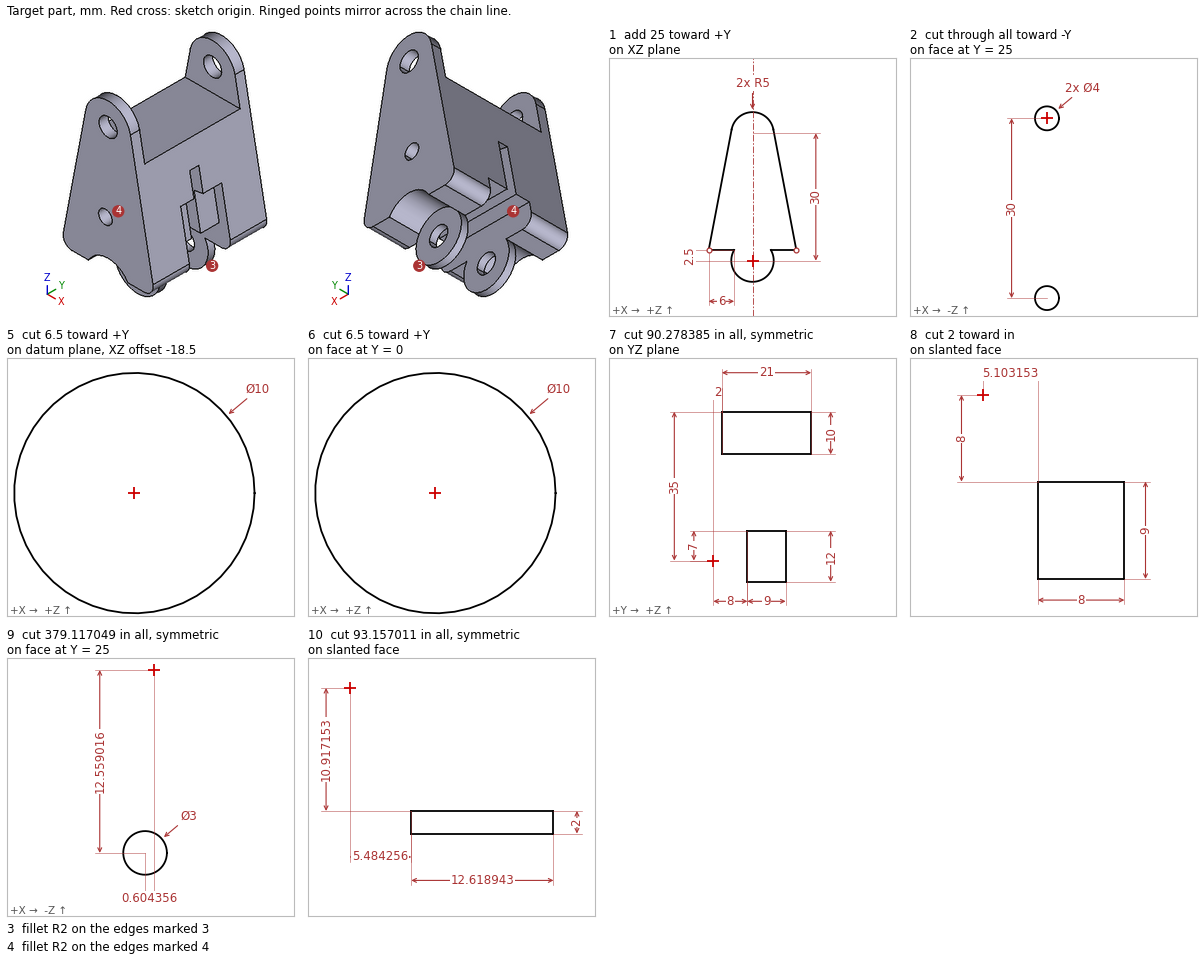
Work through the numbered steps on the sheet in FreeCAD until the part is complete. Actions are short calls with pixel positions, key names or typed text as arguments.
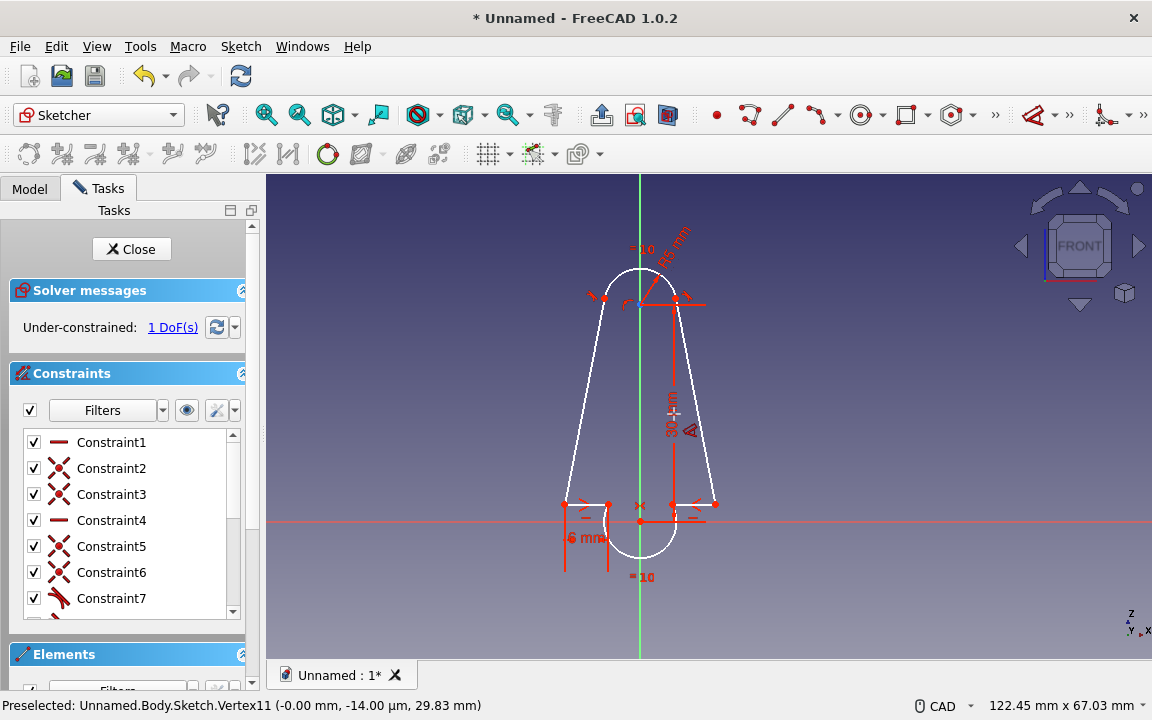
scroll(608, 505, up, 4)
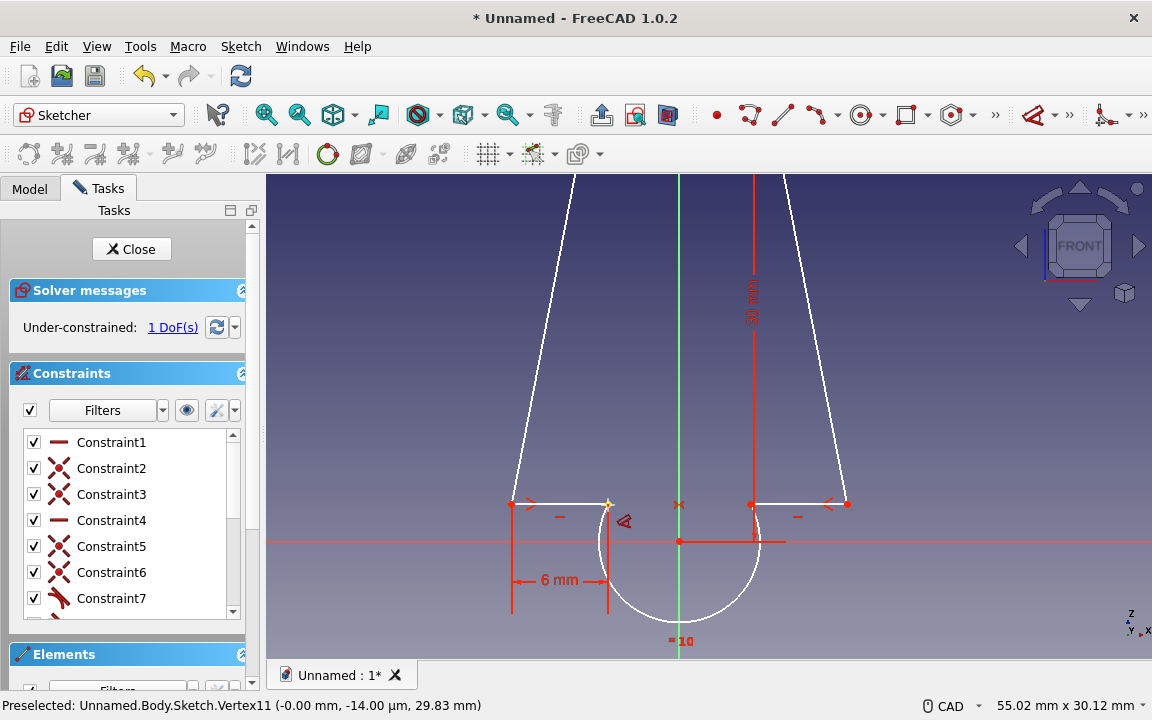
click(608, 504)
click(574, 523)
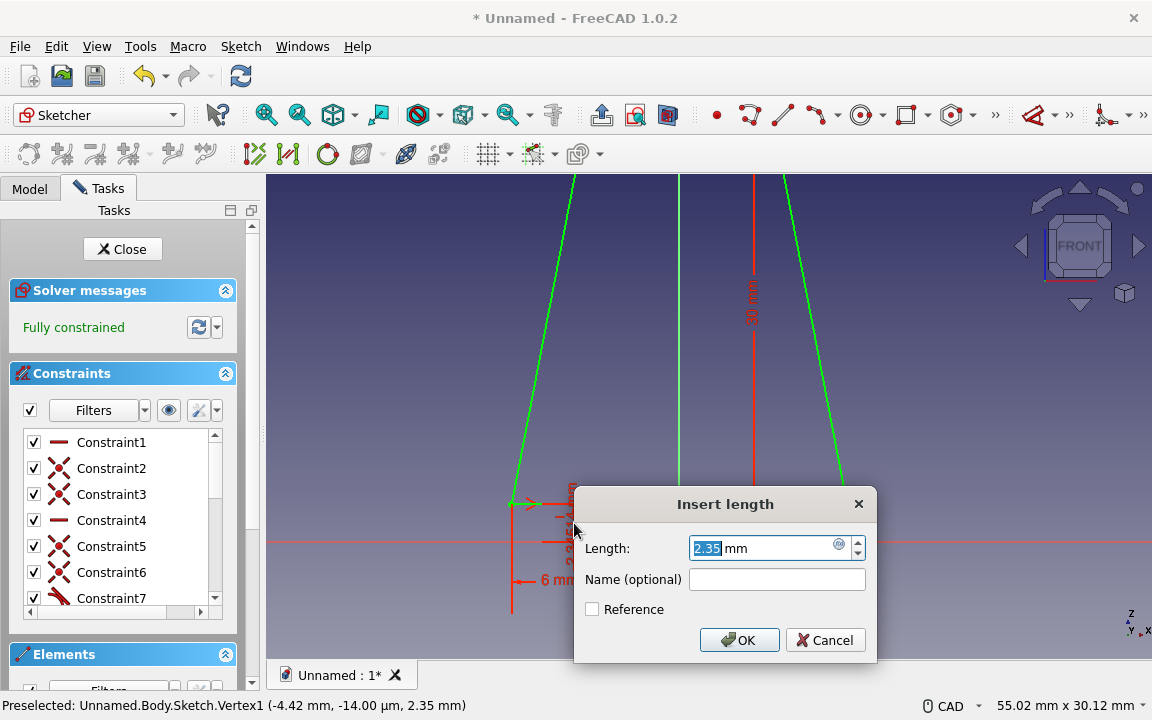
text(2.5)
key(Return)
key(Escape)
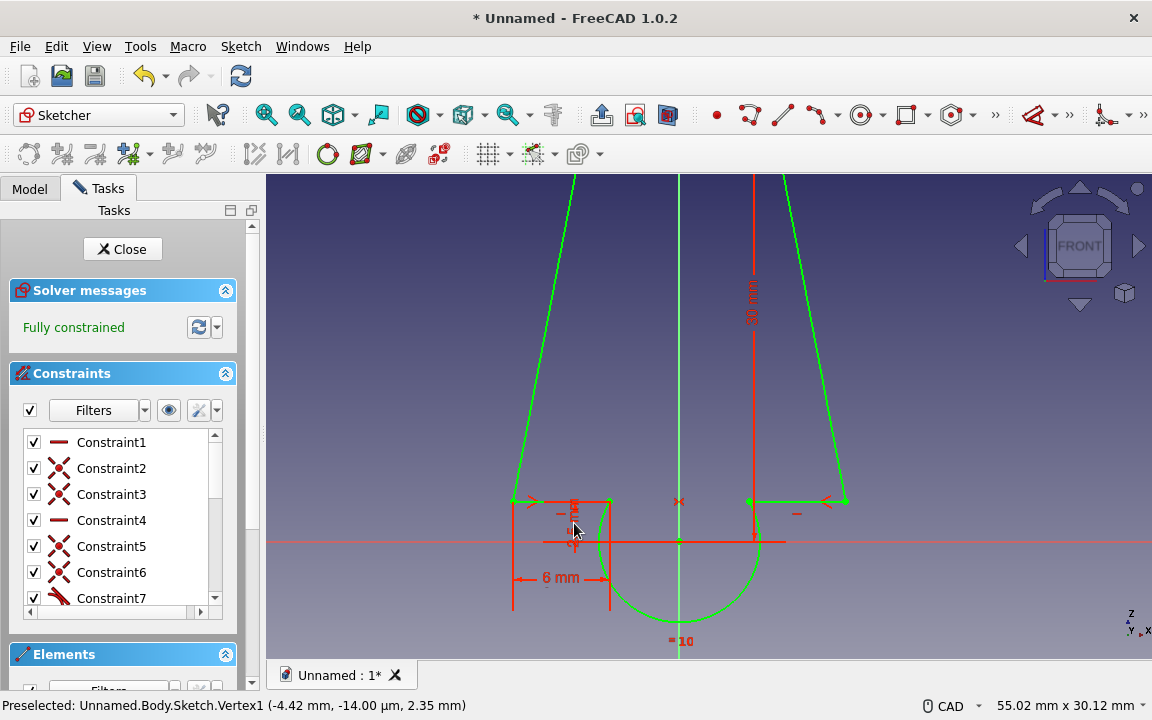
click(123, 249)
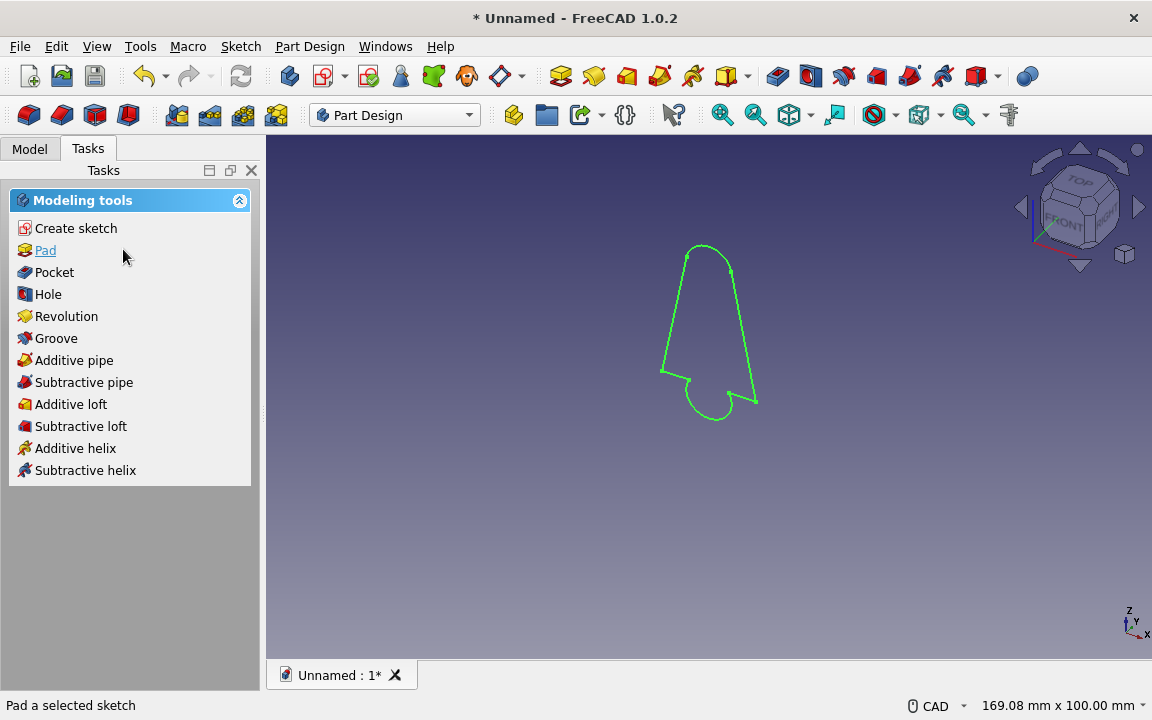
click(561, 76)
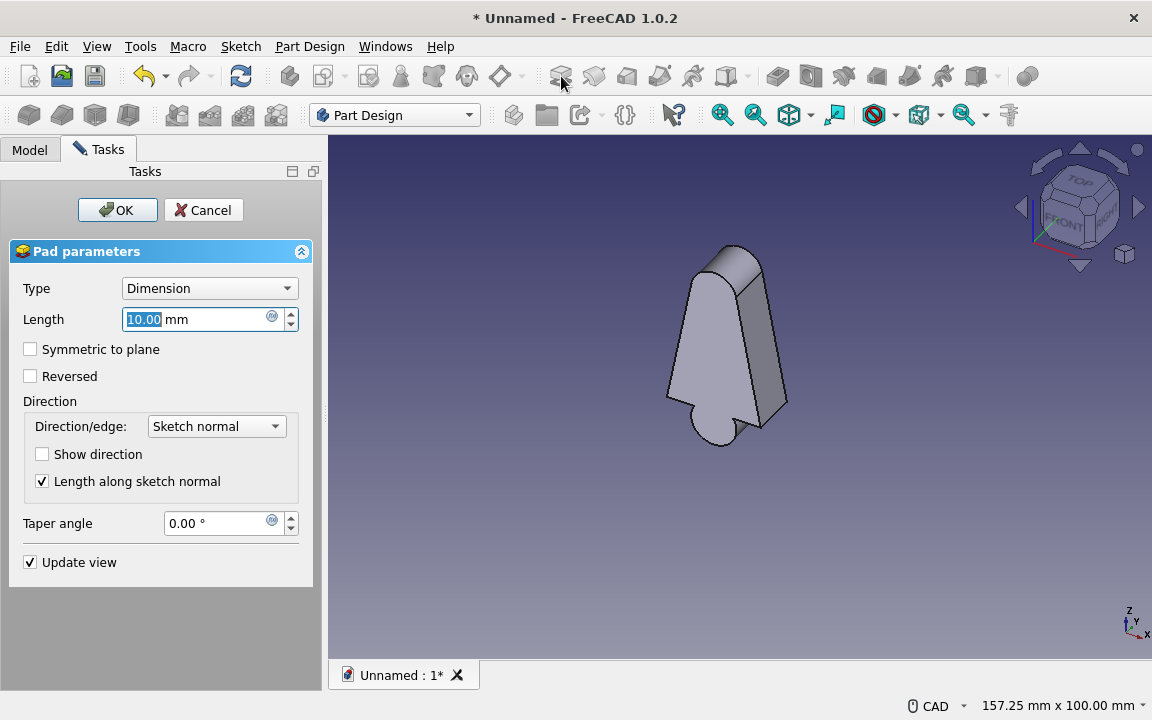
text(25)
key(Tab)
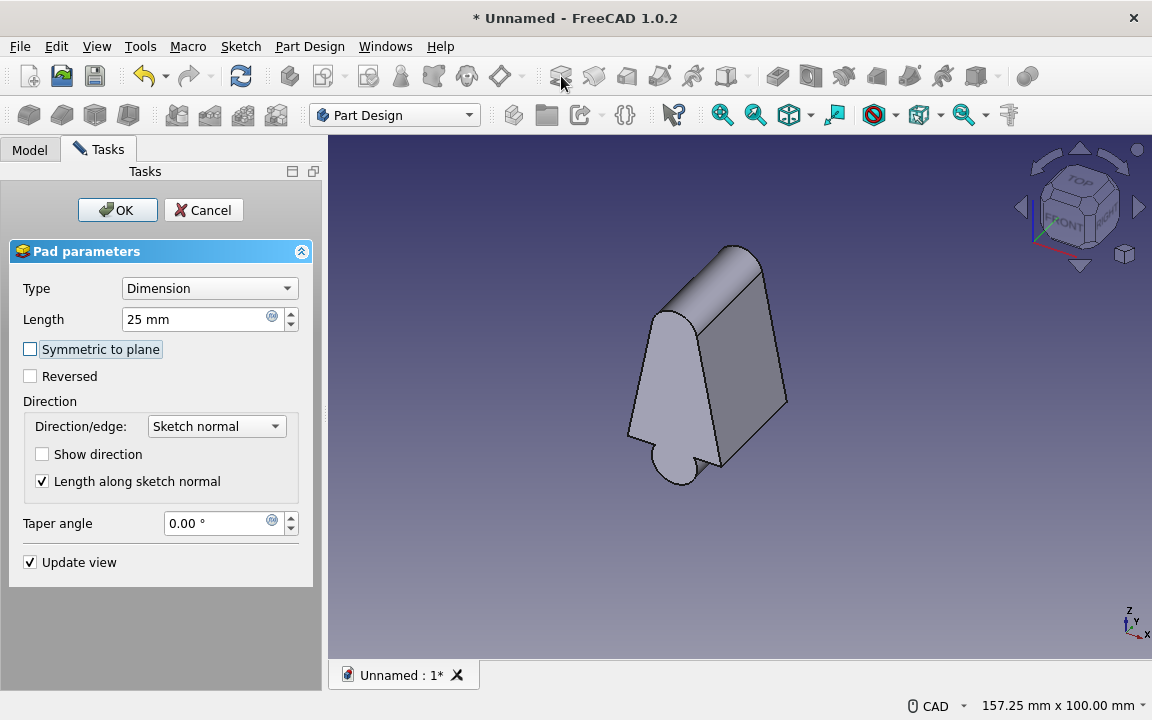
click(31, 376)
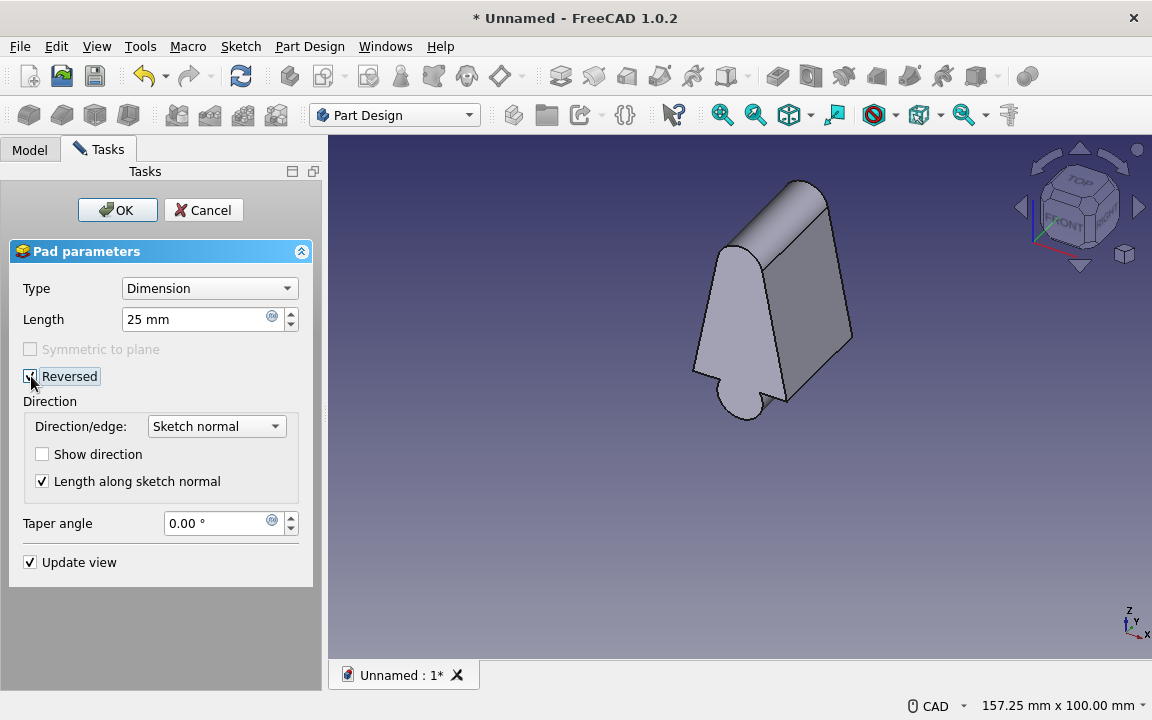
click(118, 210)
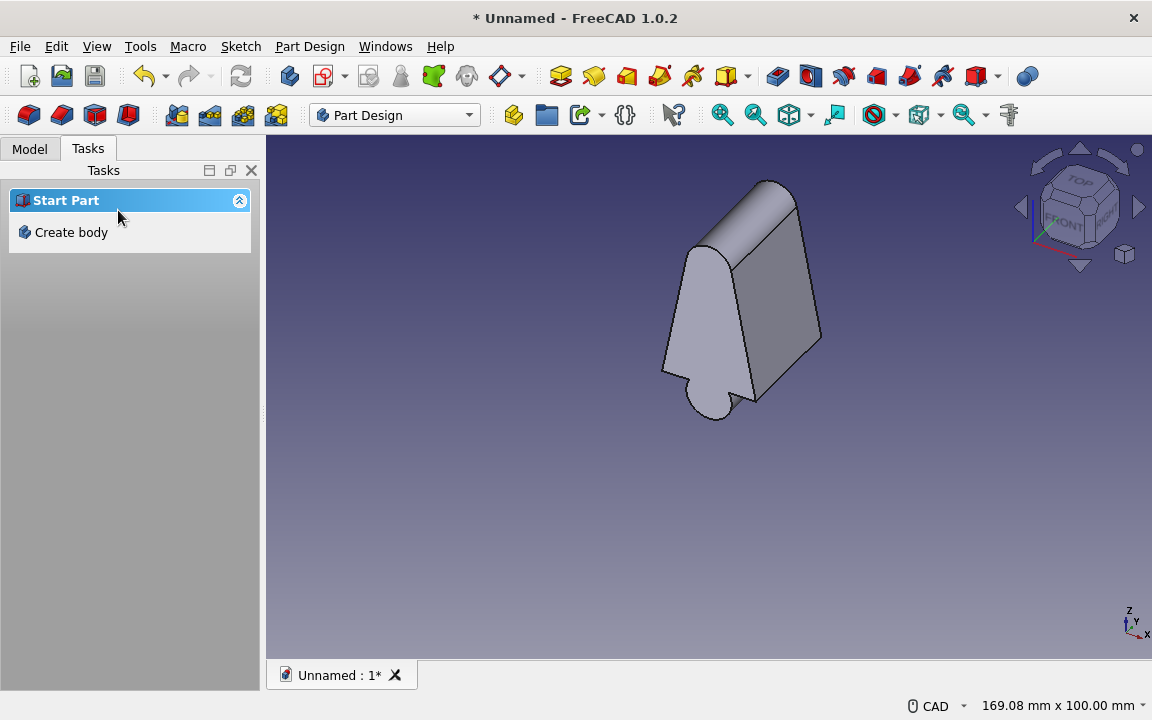
key(4)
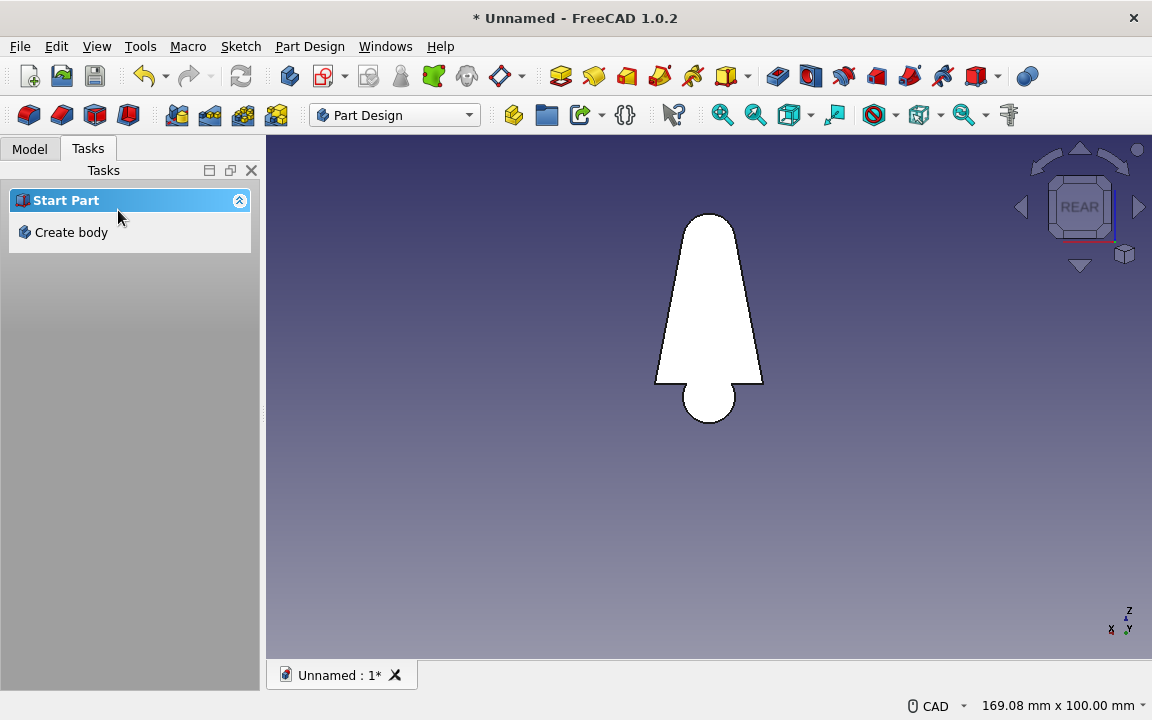
key(v)
key(f)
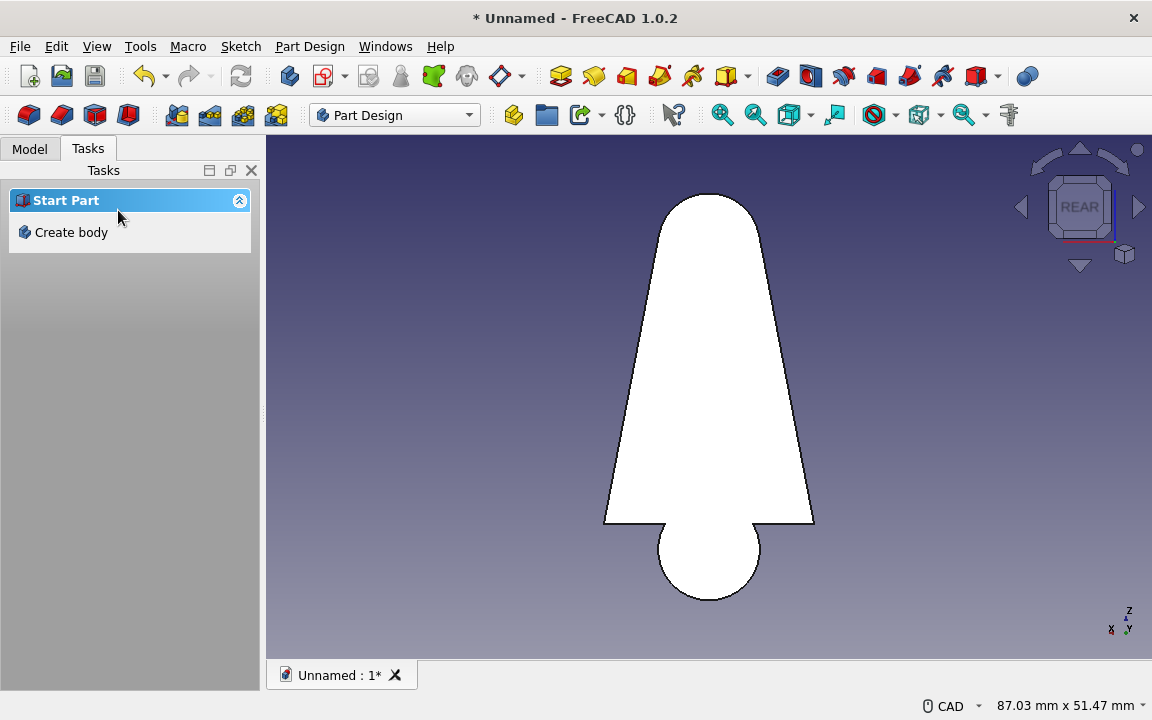
click(709, 454)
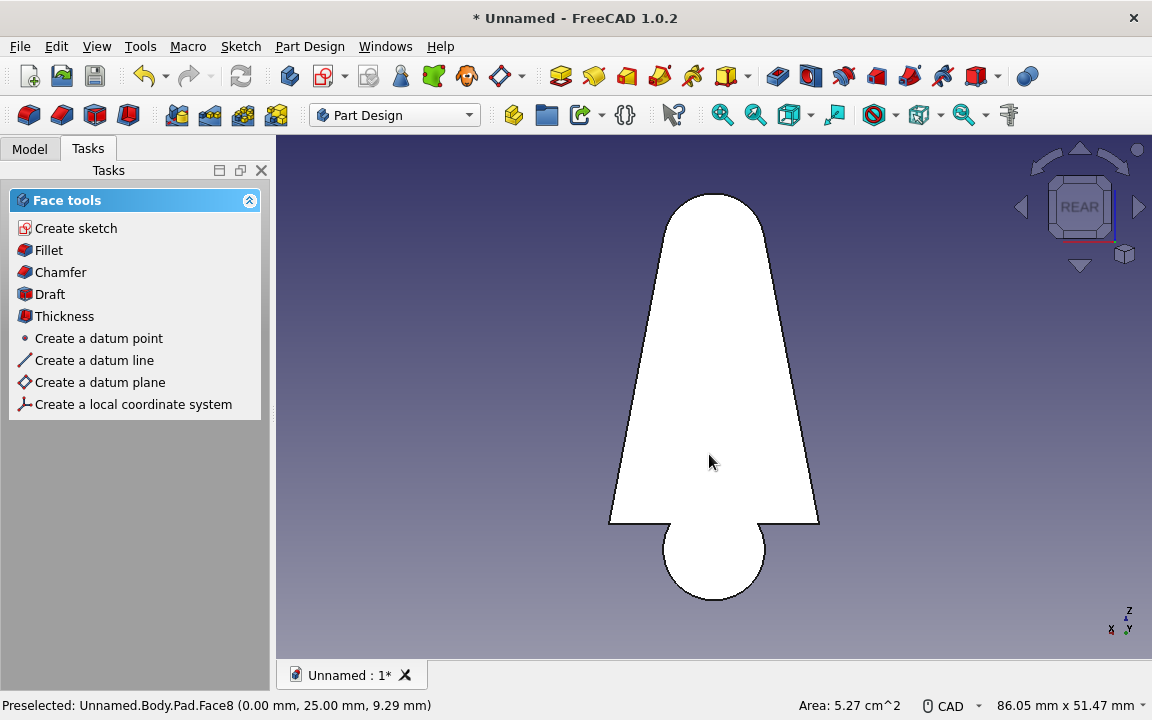
click(322, 76)